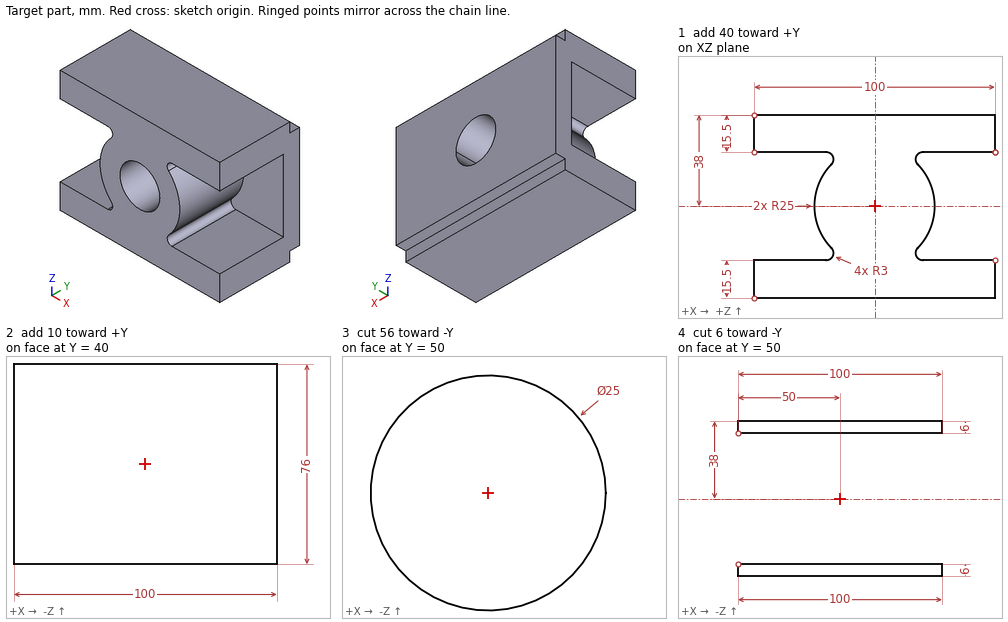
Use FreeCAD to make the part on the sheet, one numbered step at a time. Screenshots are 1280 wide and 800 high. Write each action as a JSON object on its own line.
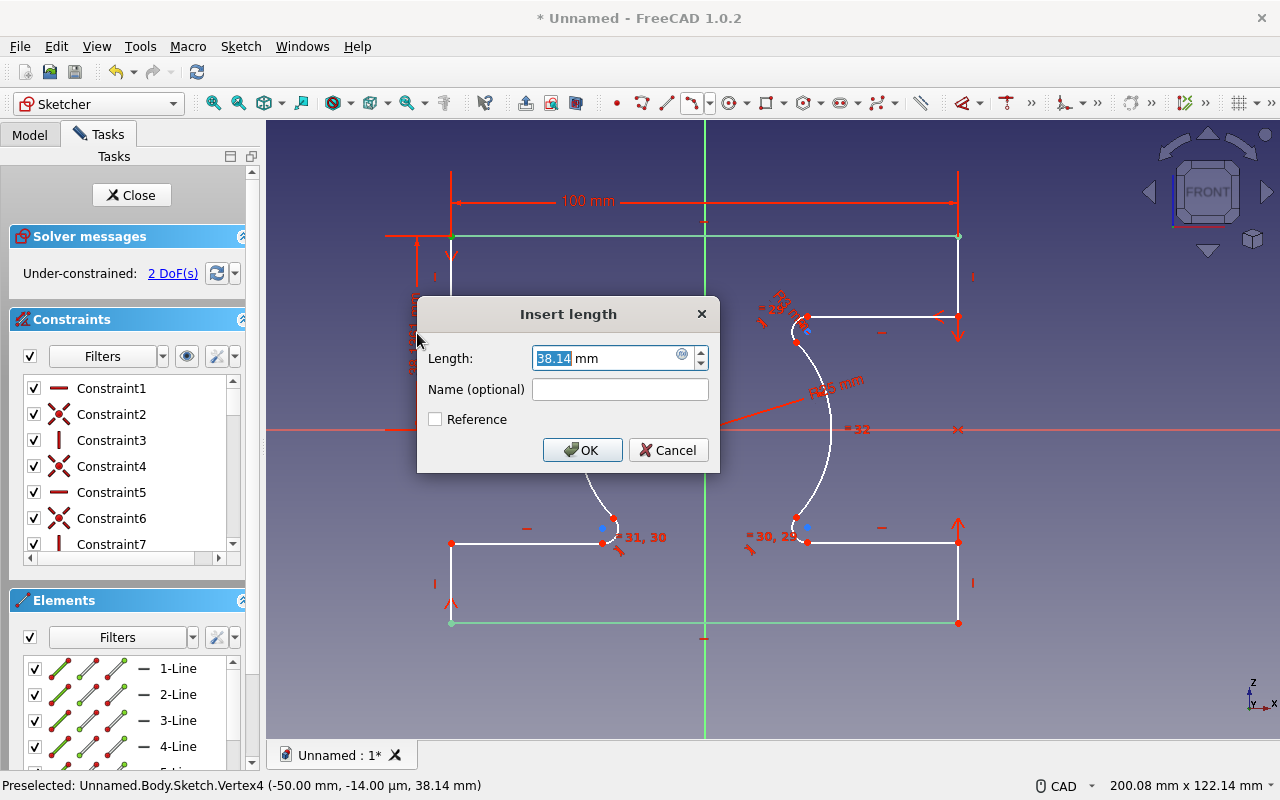
{"action": "type", "text": "38"}
{"action": "key", "text": "Return"}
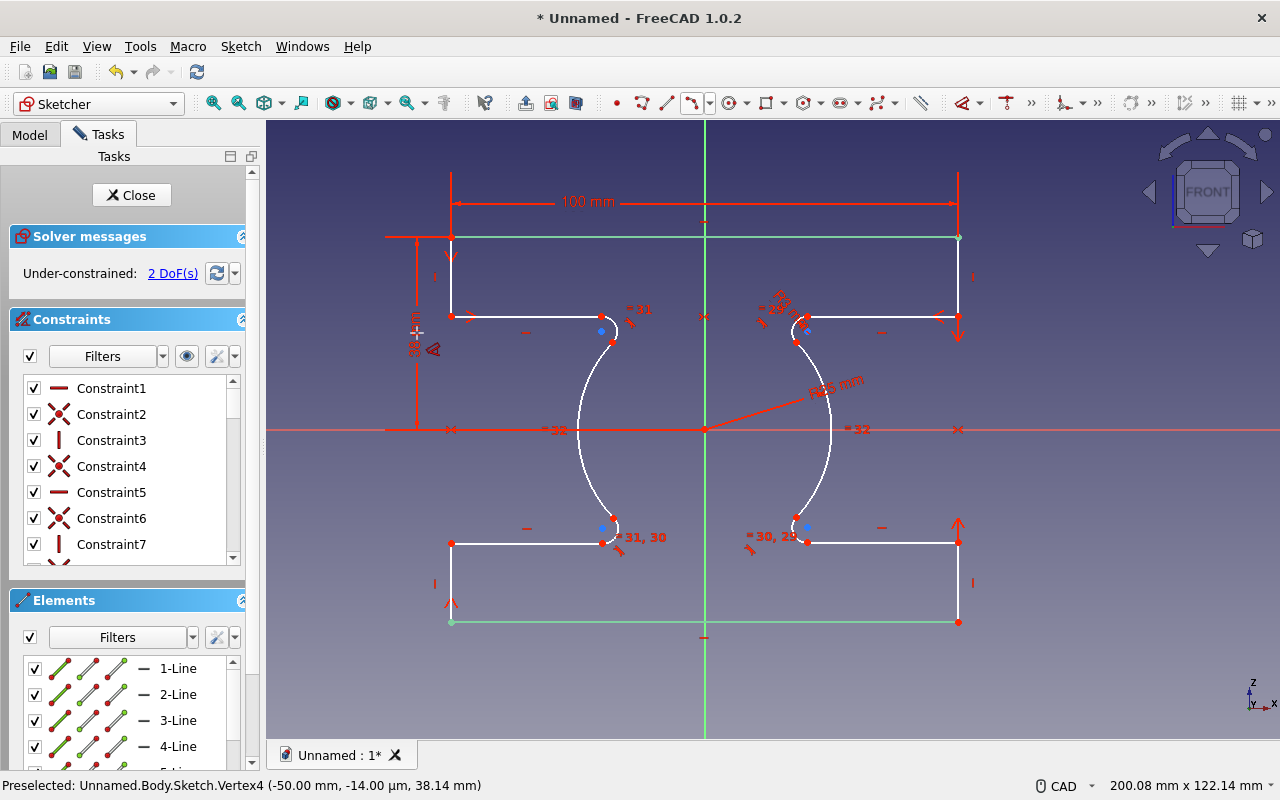
{"action": "left_click", "coordinate": [451, 293]}
{"action": "left_click", "coordinate": [417, 277]}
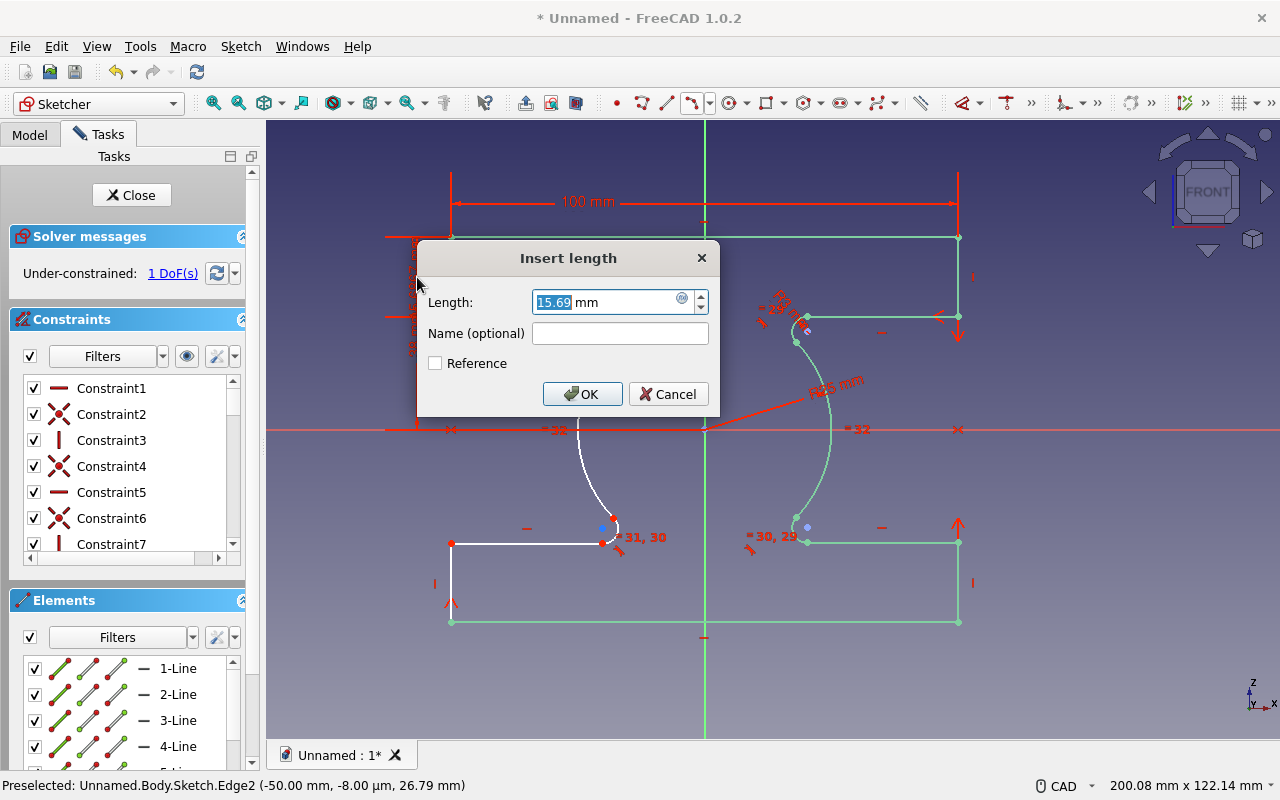
{"action": "type", "text": "15.5"}
{"action": "key", "text": "Return"}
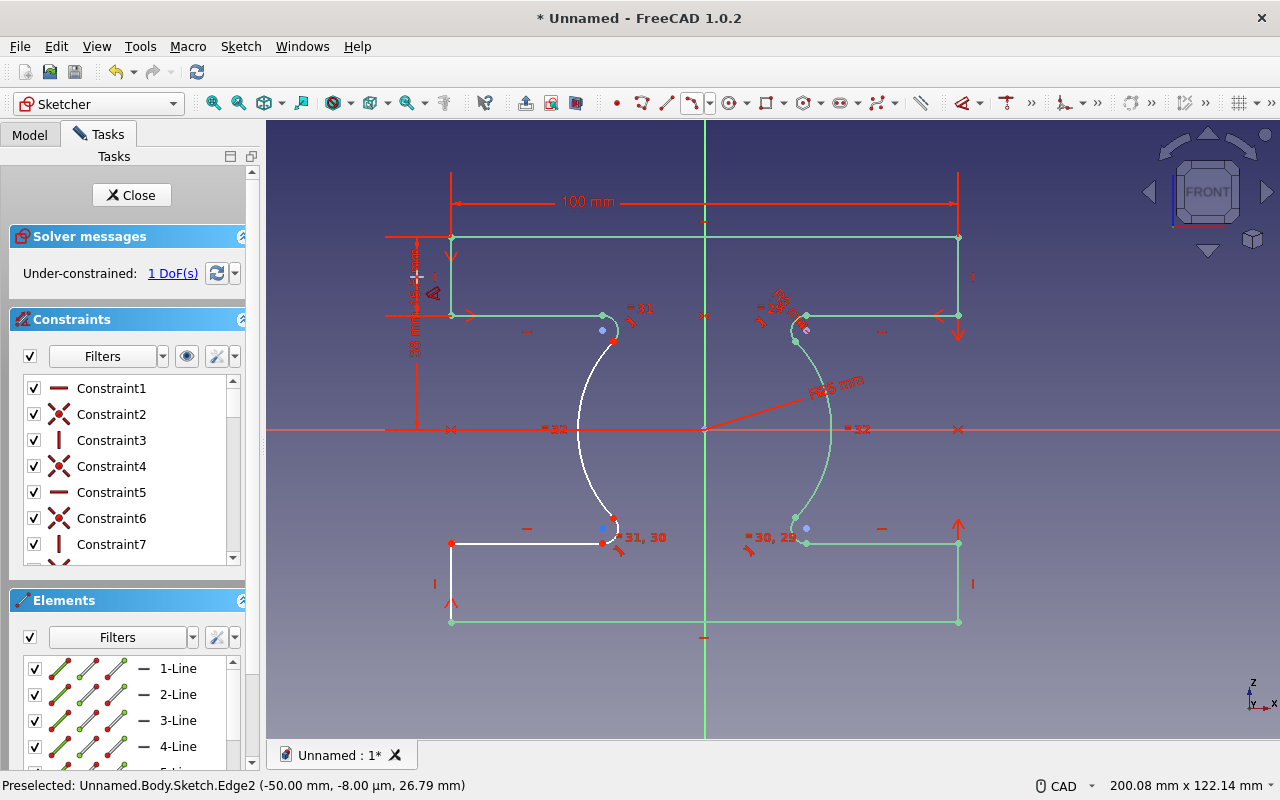
{"action": "left_click", "coordinate": [451, 599]}
{"action": "left_click", "coordinate": [417, 583]}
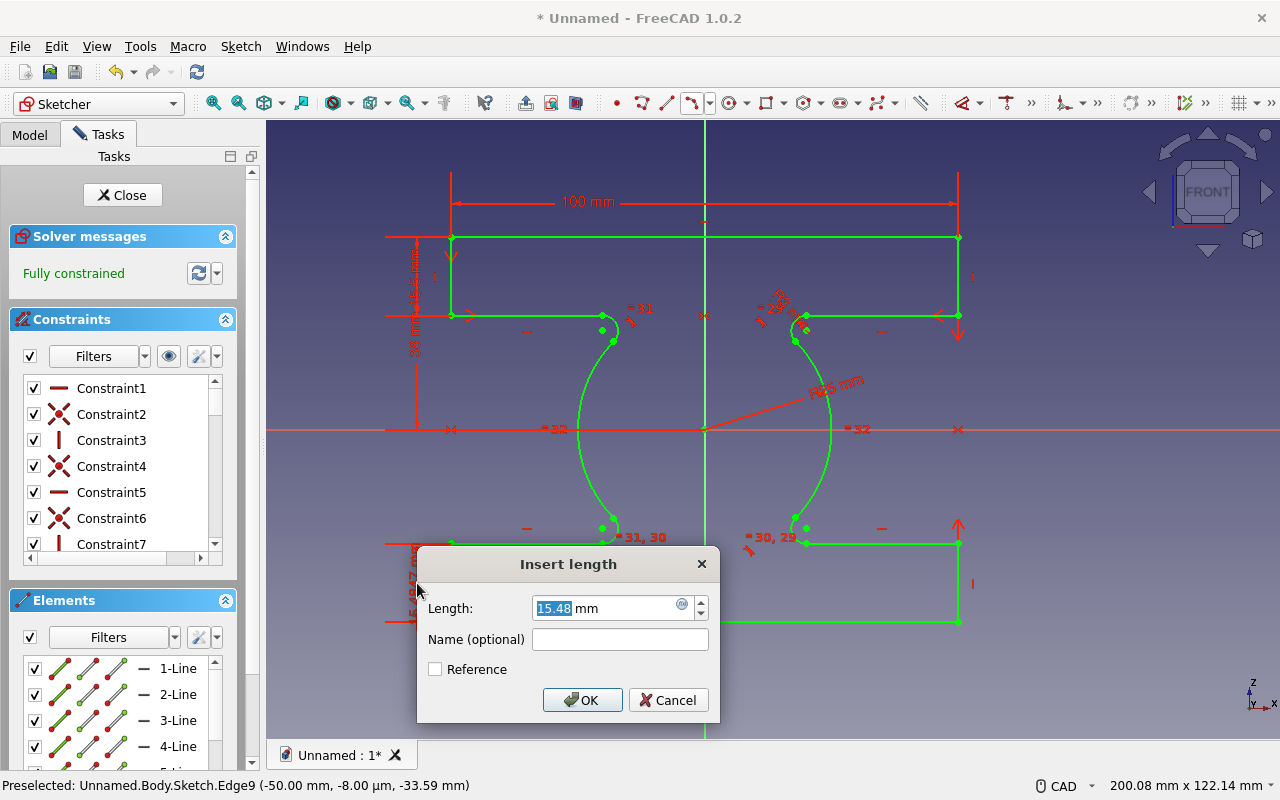
{"action": "type", "text": "15.5"}
{"action": "key", "text": "Return"}
{"action": "key", "text": "Escape"}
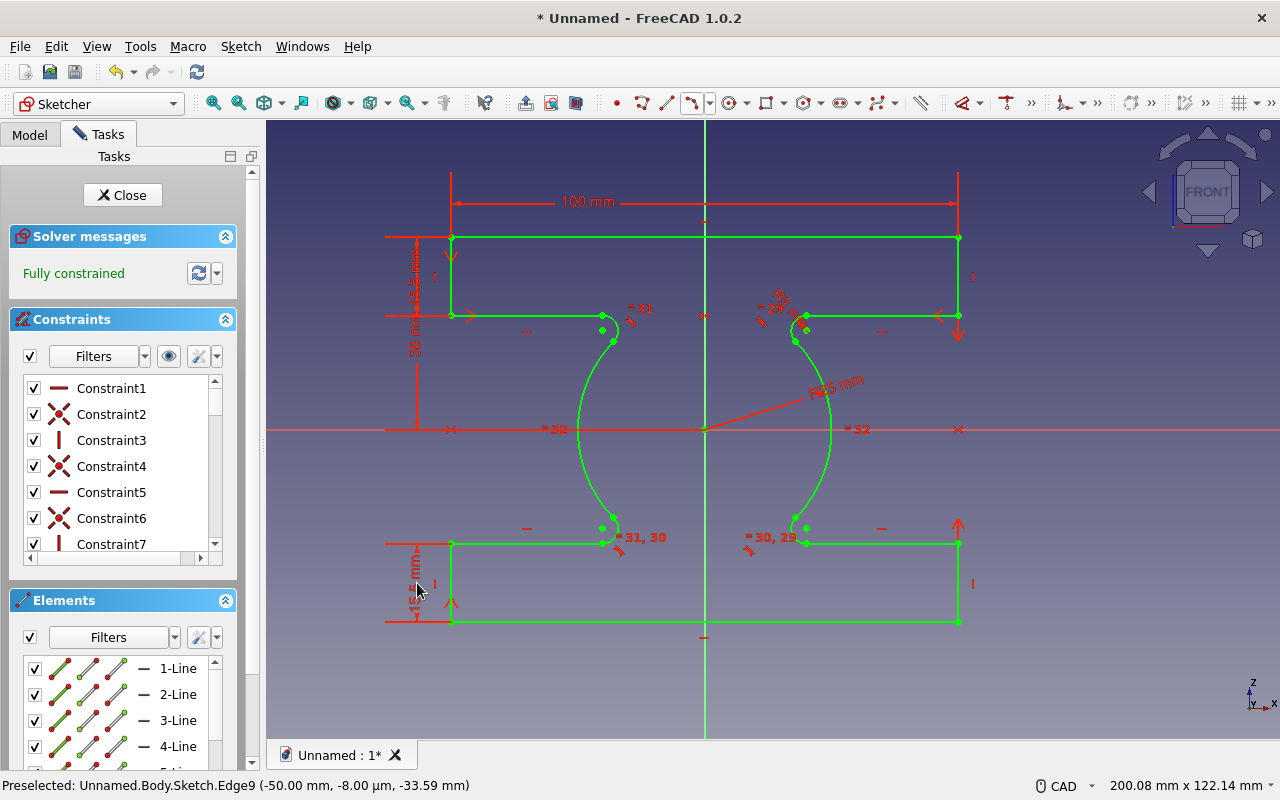
{"action": "left_click", "coordinate": [123, 195]}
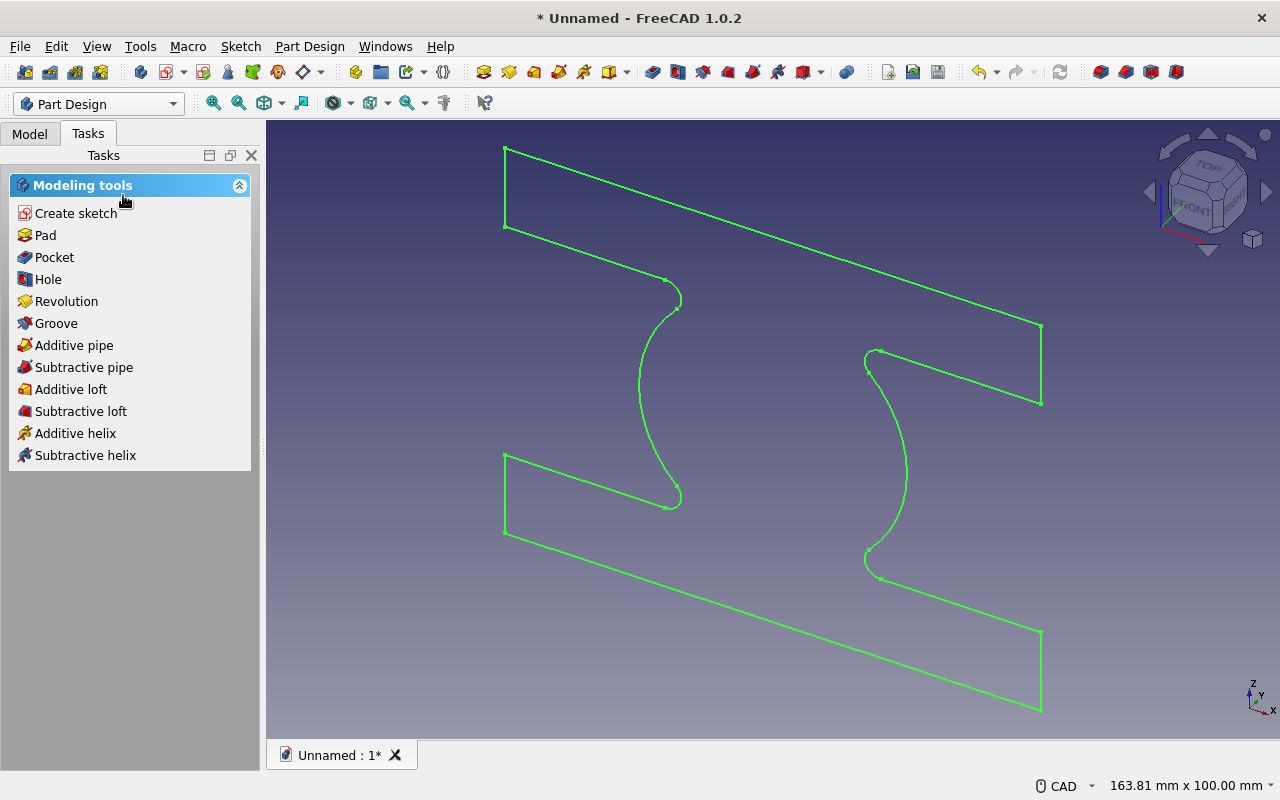
{"action": "left_click", "coordinate": [484, 72]}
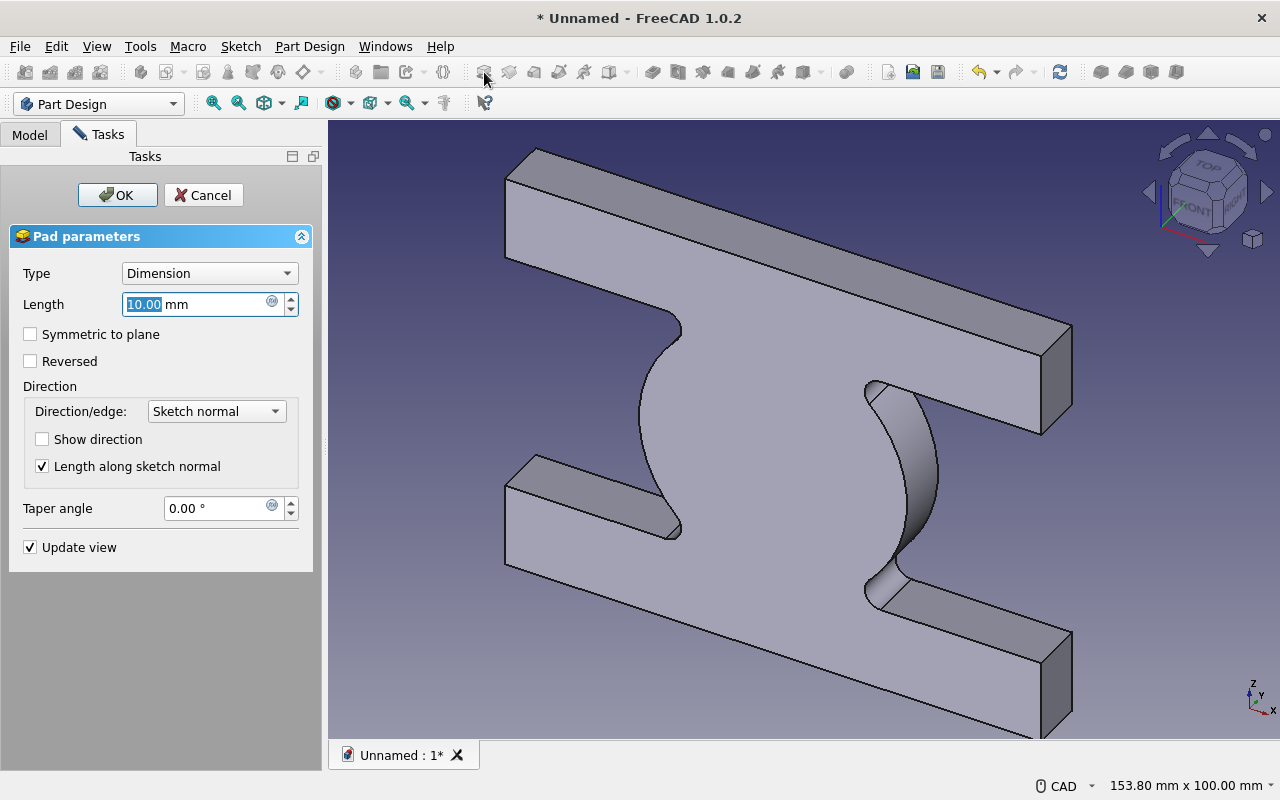
{"action": "type", "text": "40"}
{"action": "key", "text": "Tab"}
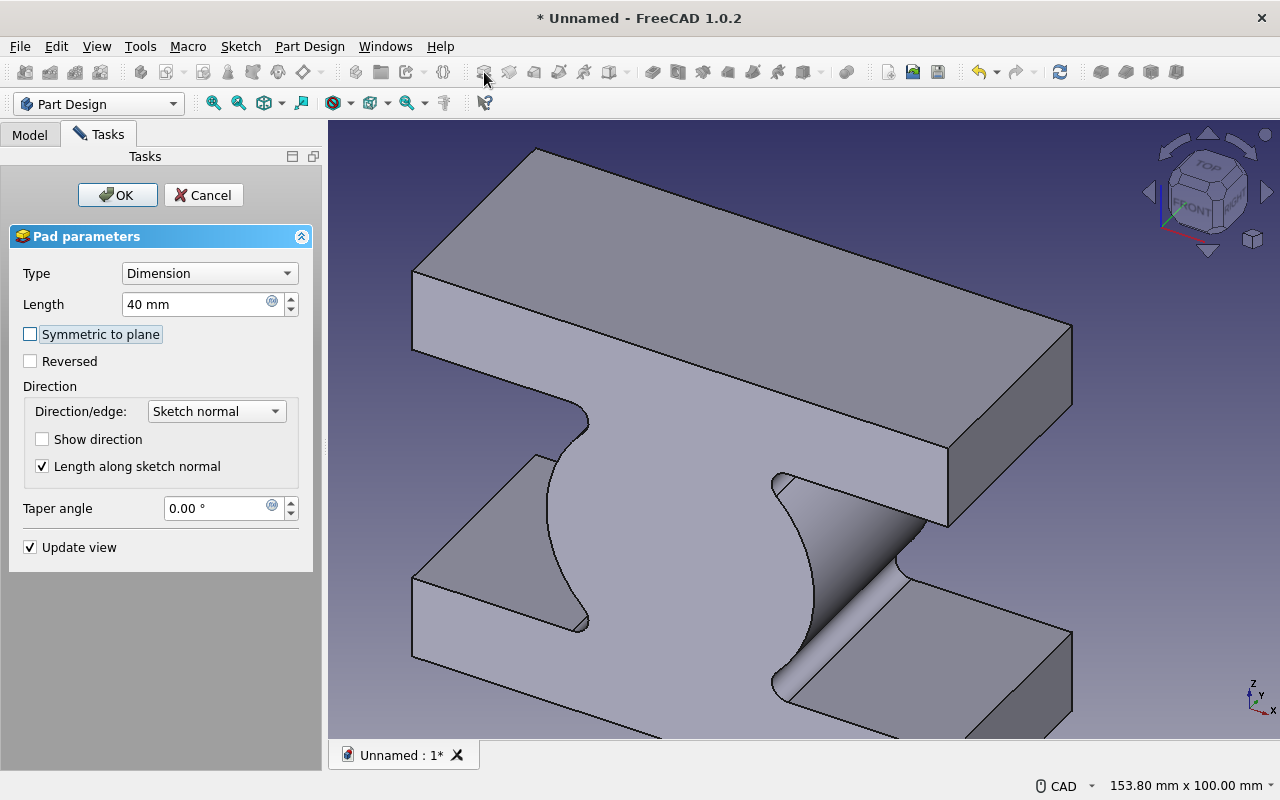
{"action": "left_click", "coordinate": [31, 361]}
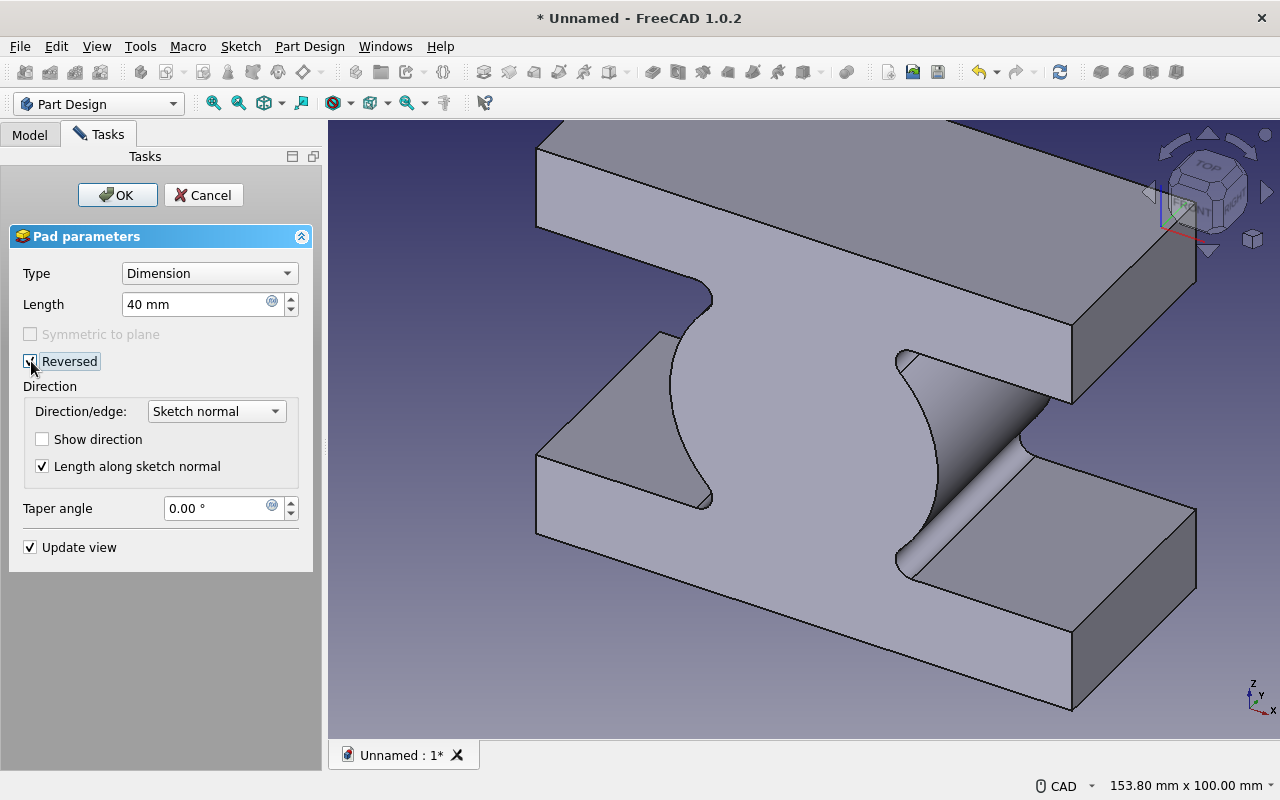
{"action": "left_click", "coordinate": [118, 195]}